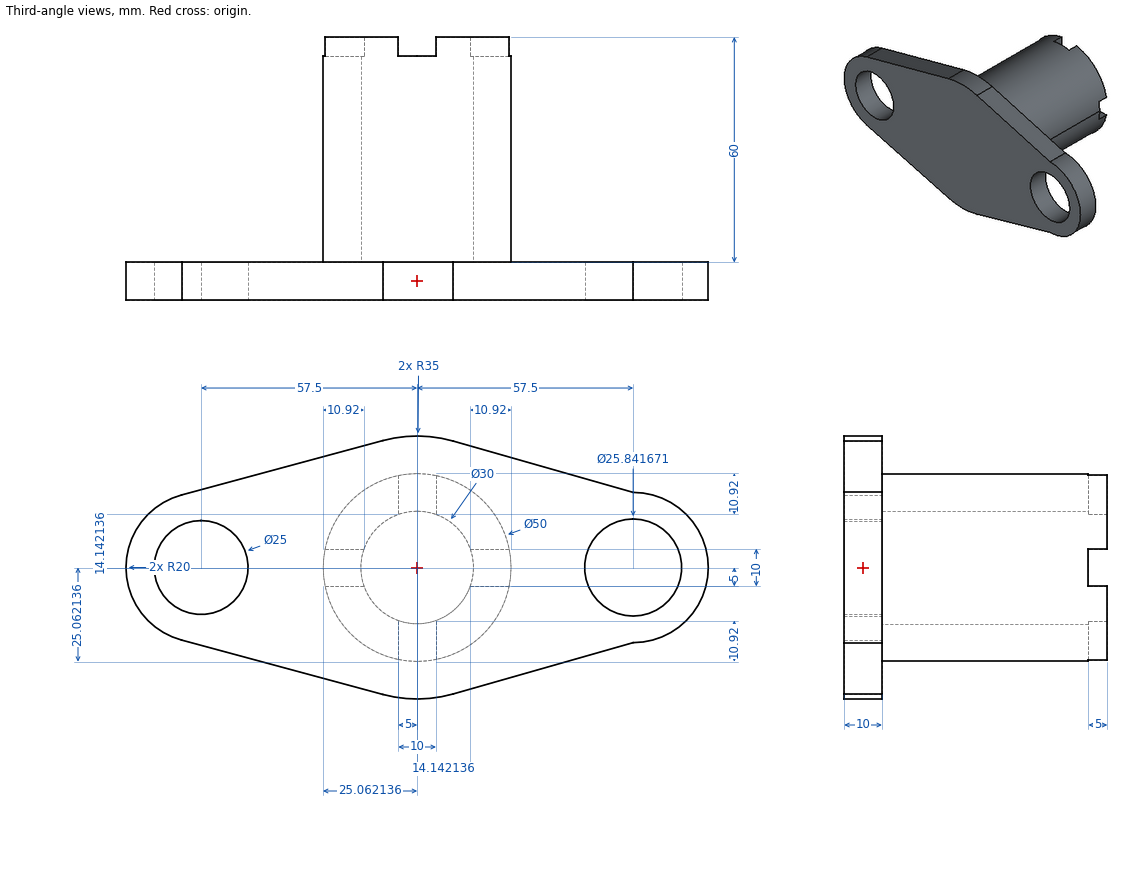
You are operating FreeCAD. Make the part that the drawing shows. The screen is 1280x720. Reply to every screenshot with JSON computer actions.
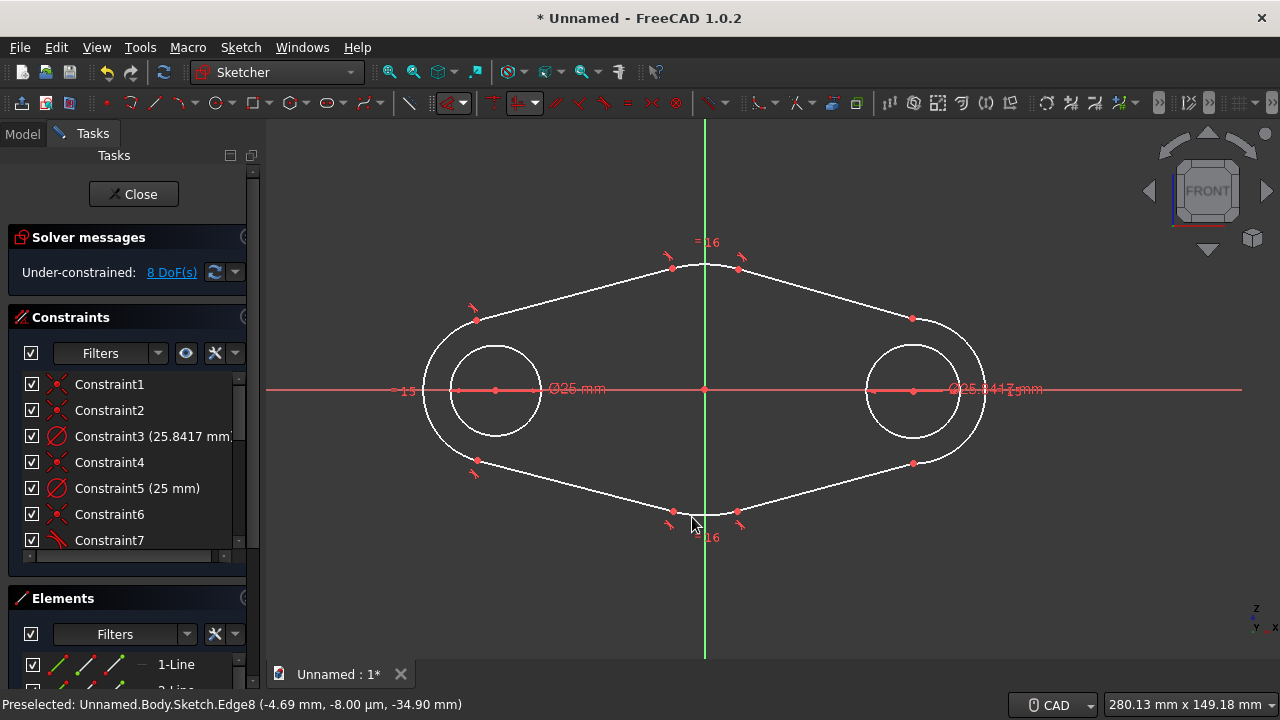
{"action": "left_click", "coordinate": [496, 391]}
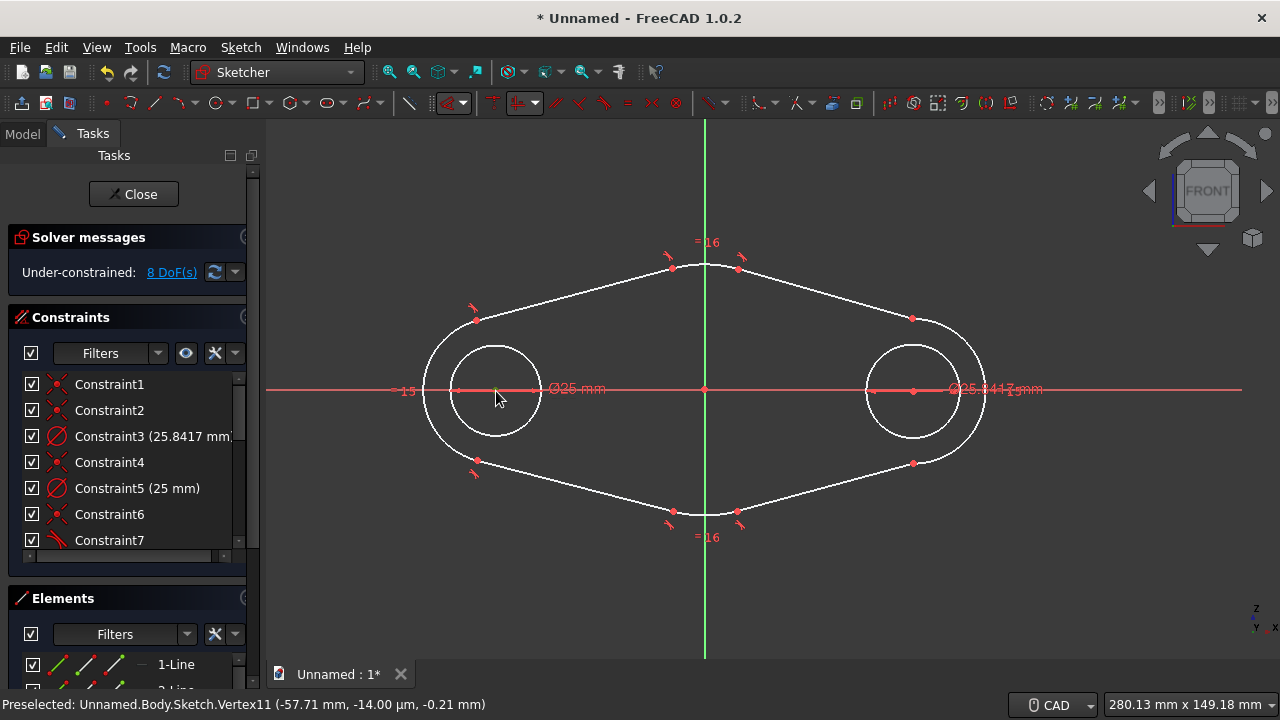
{"action": "left_click", "coordinate": [353, 390]}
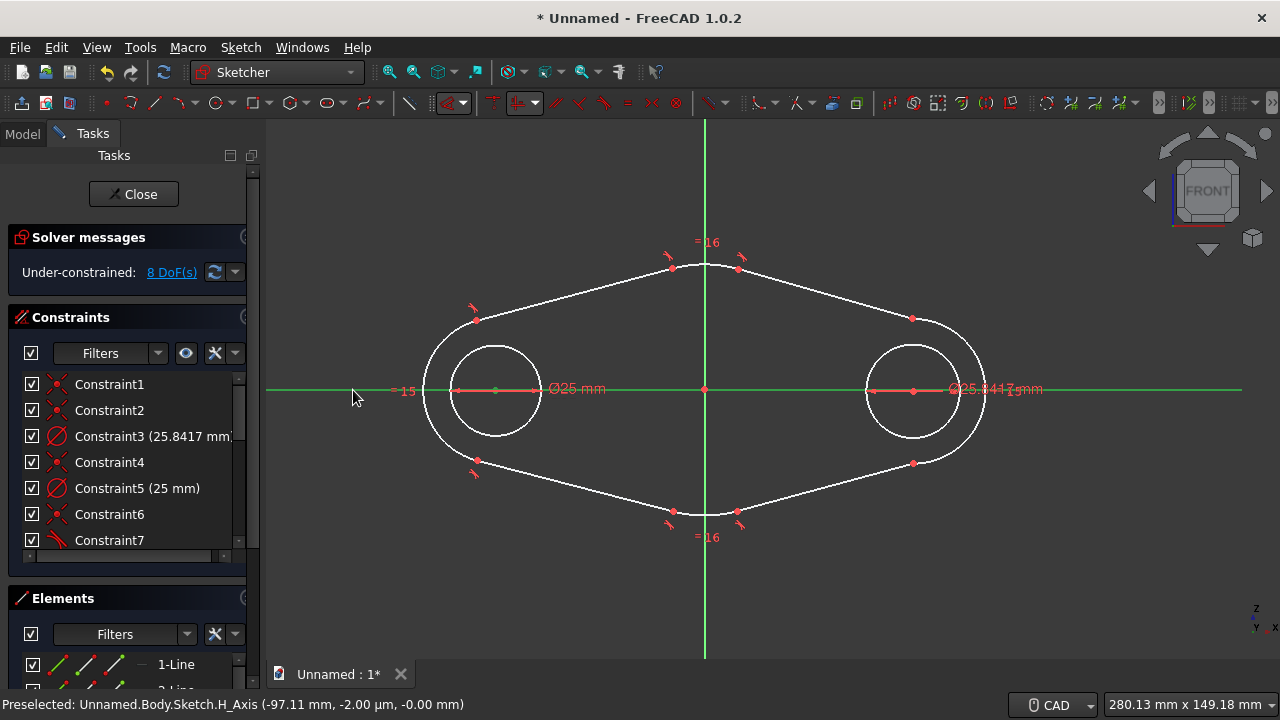
{"action": "left_click", "coordinate": [494, 104]}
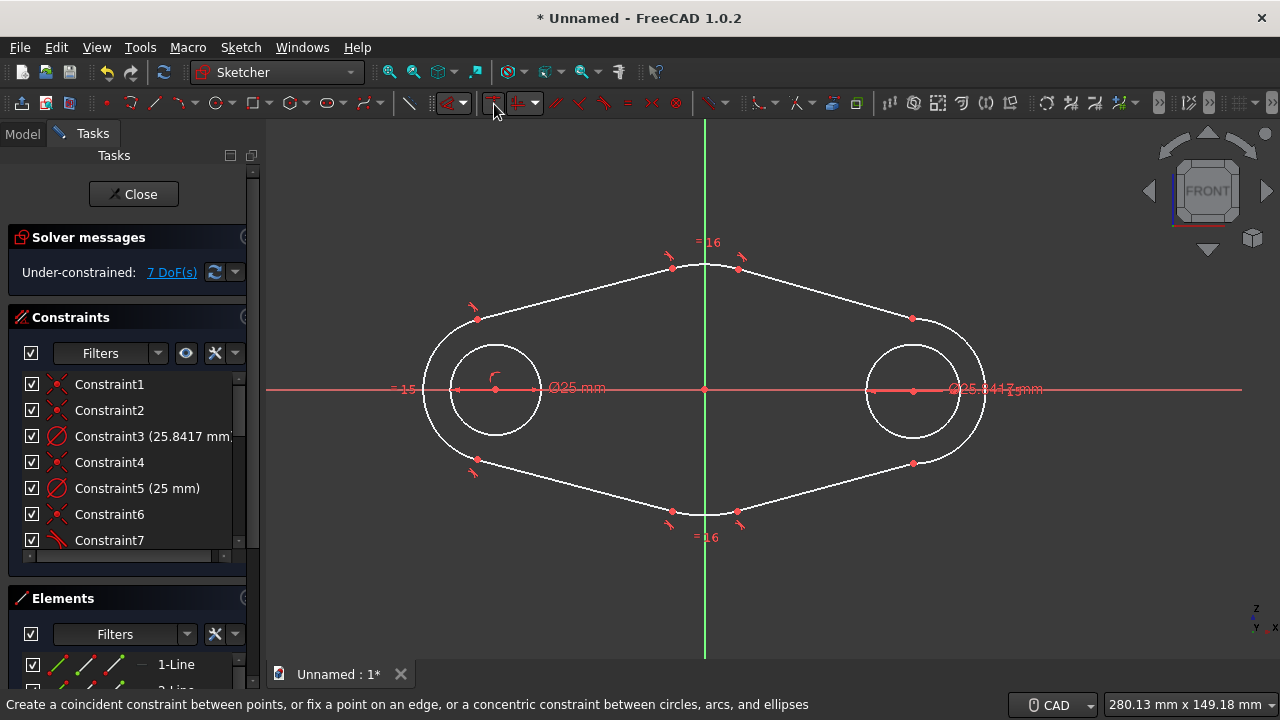
{"action": "left_click", "coordinate": [913, 391]}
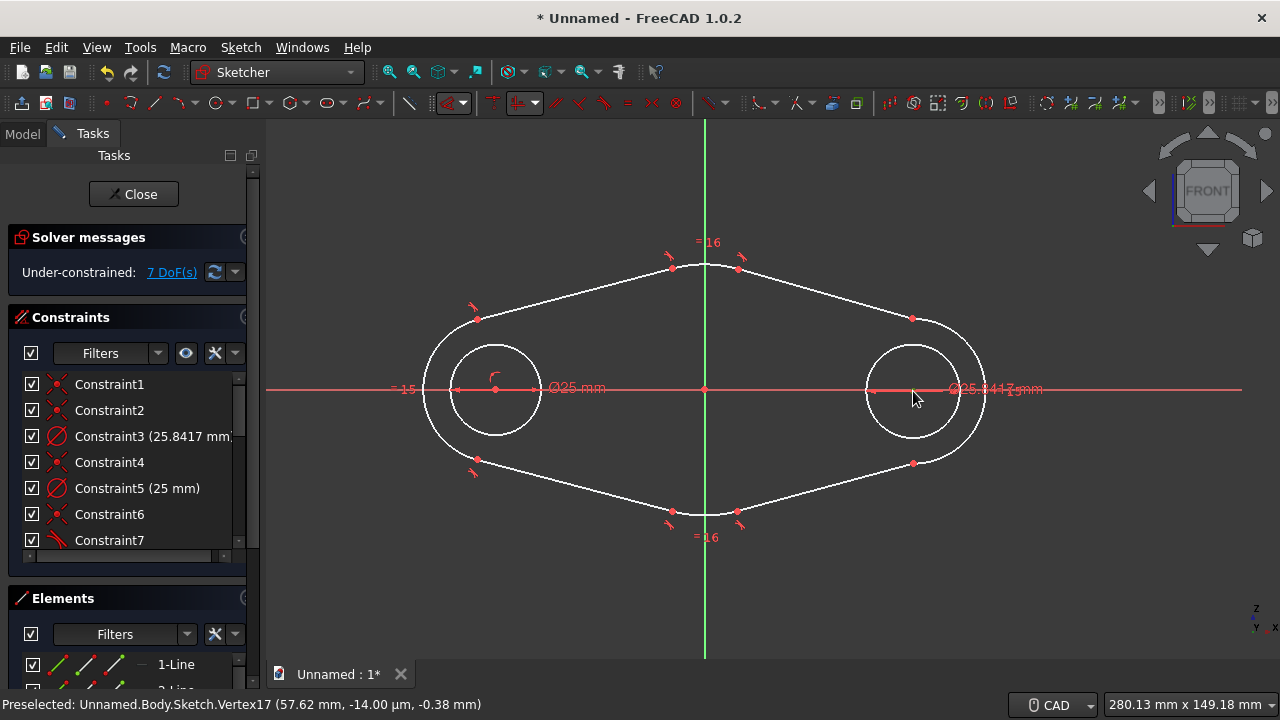
{"action": "left_click", "coordinate": [353, 390]}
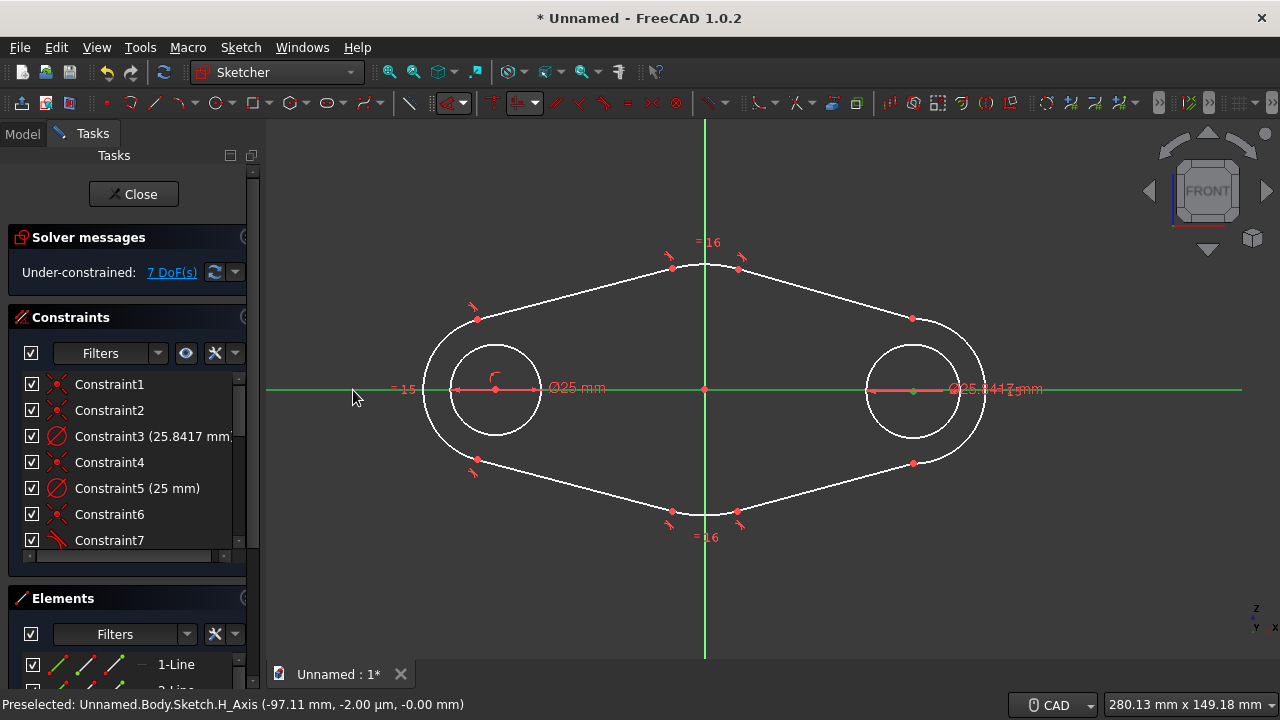
{"action": "key", "text": "c"}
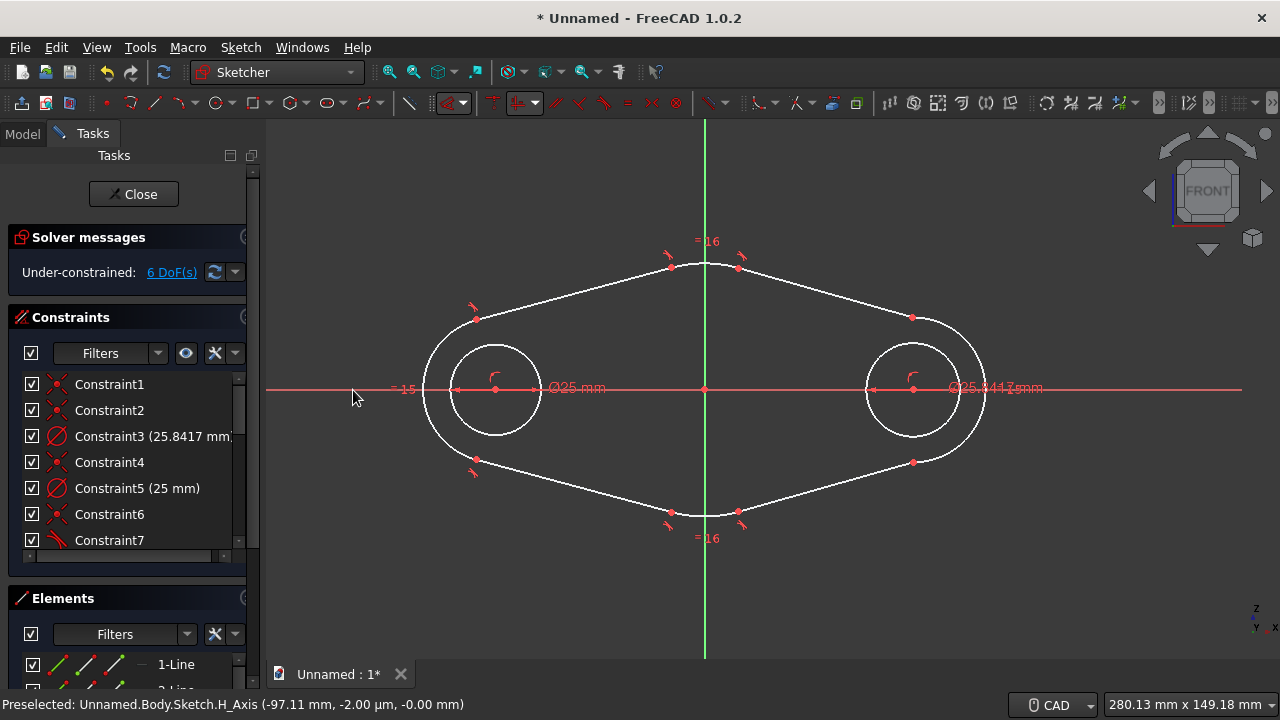
{"action": "left_click", "coordinate": [433, 354]}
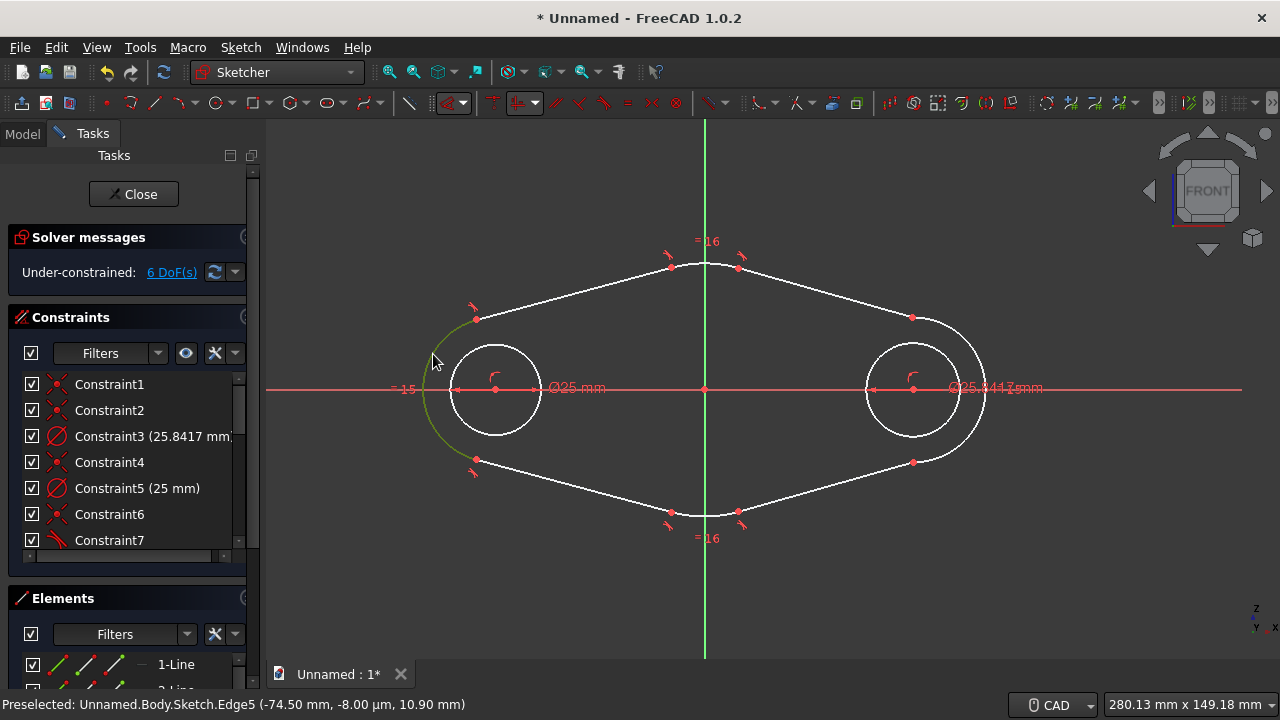
{"action": "key", "text": "k r"}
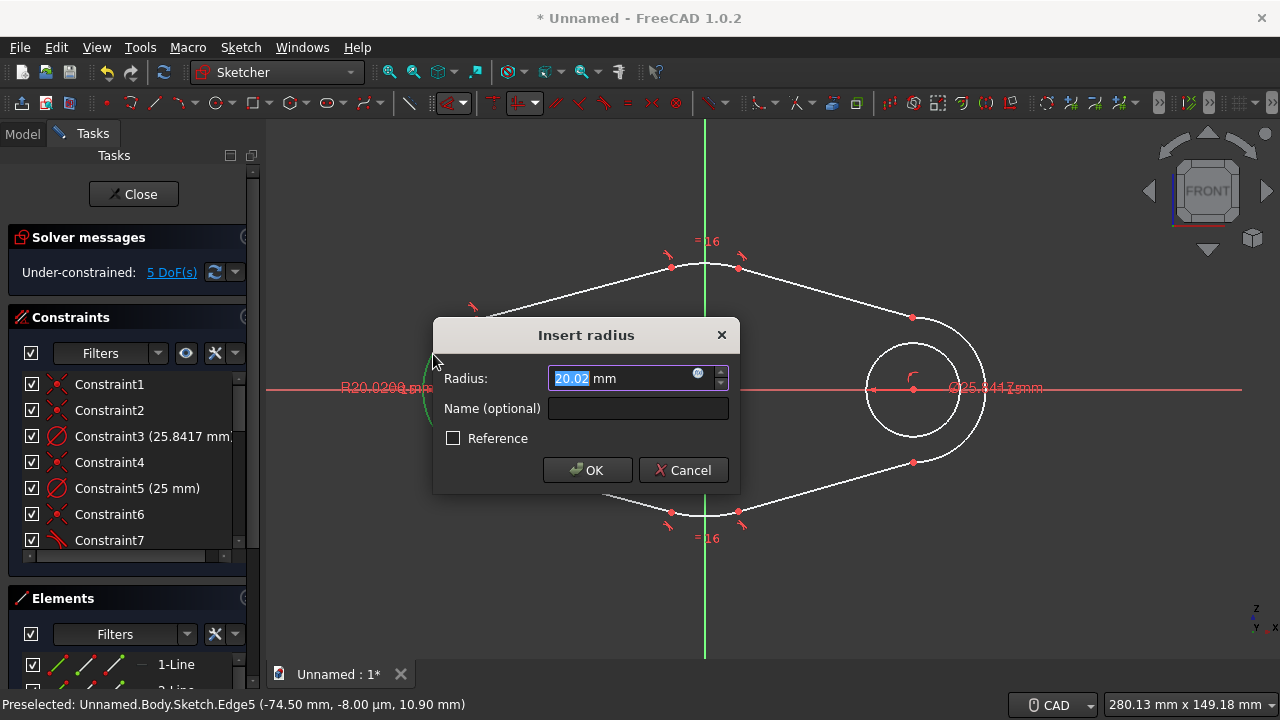
{"action": "type", "text": "20"}
{"action": "key", "text": "Return"}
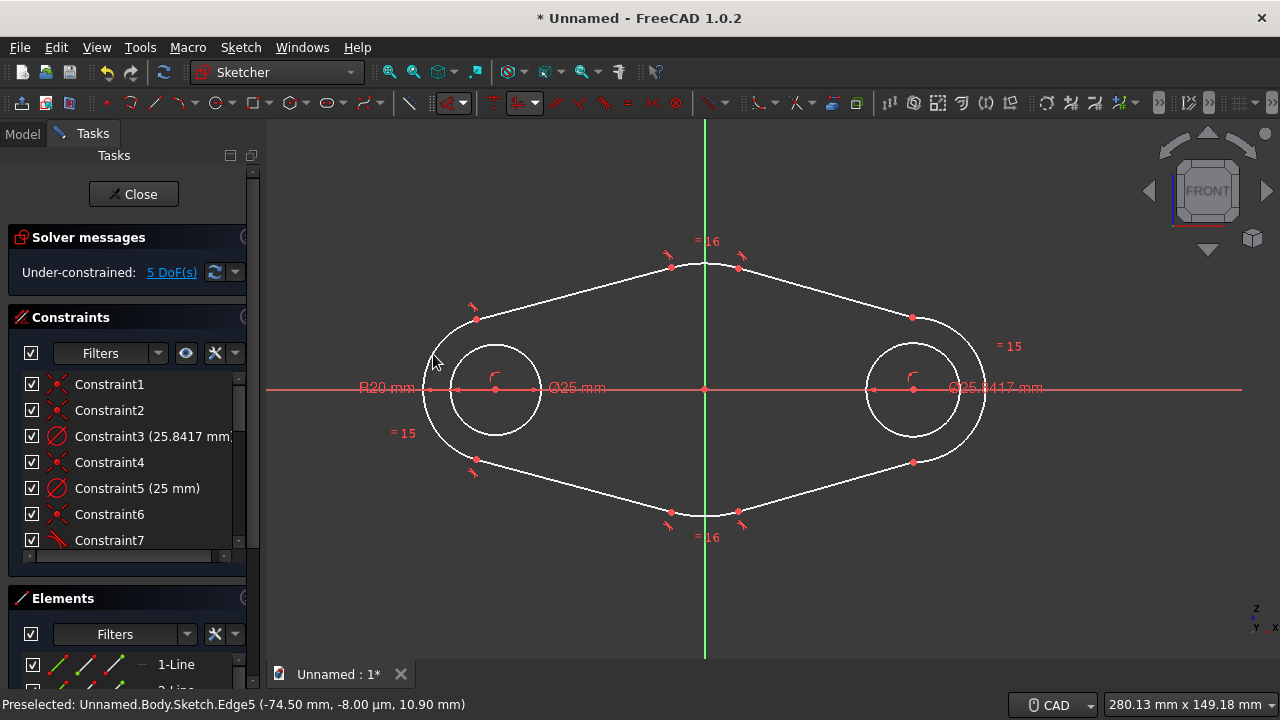
{"action": "left_click", "coordinate": [719, 264]}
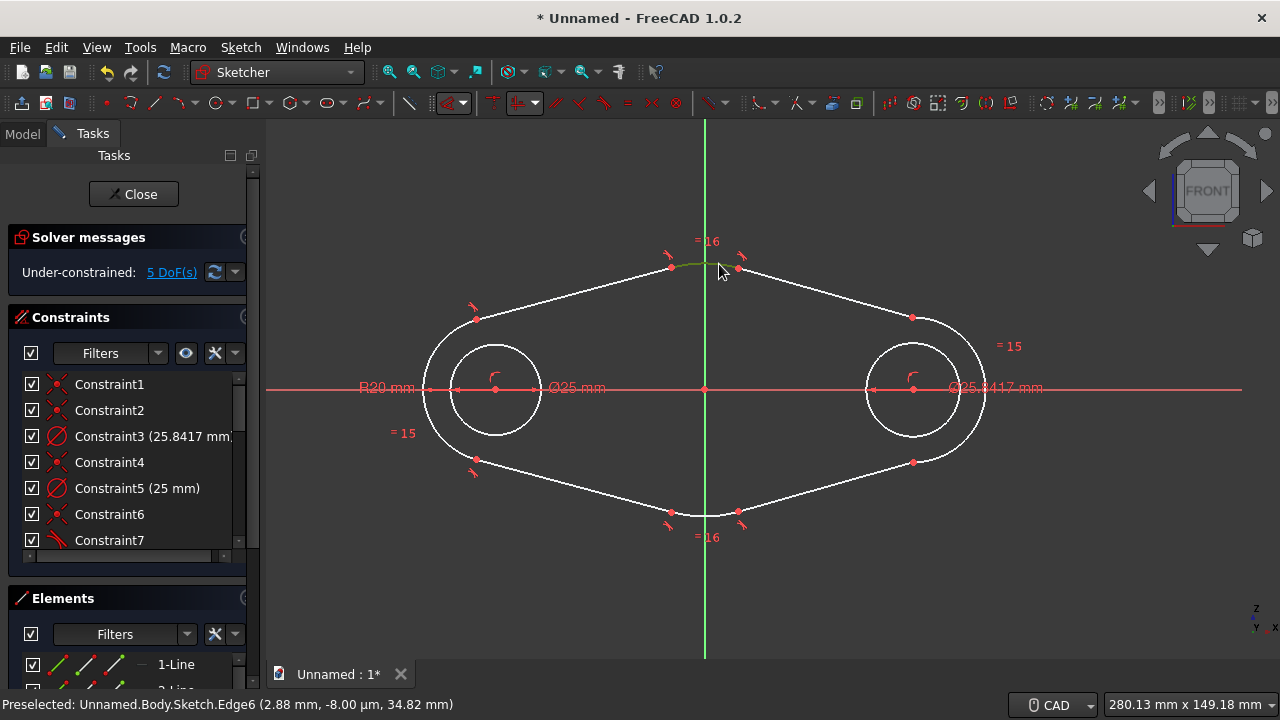
{"action": "key", "text": "k r"}